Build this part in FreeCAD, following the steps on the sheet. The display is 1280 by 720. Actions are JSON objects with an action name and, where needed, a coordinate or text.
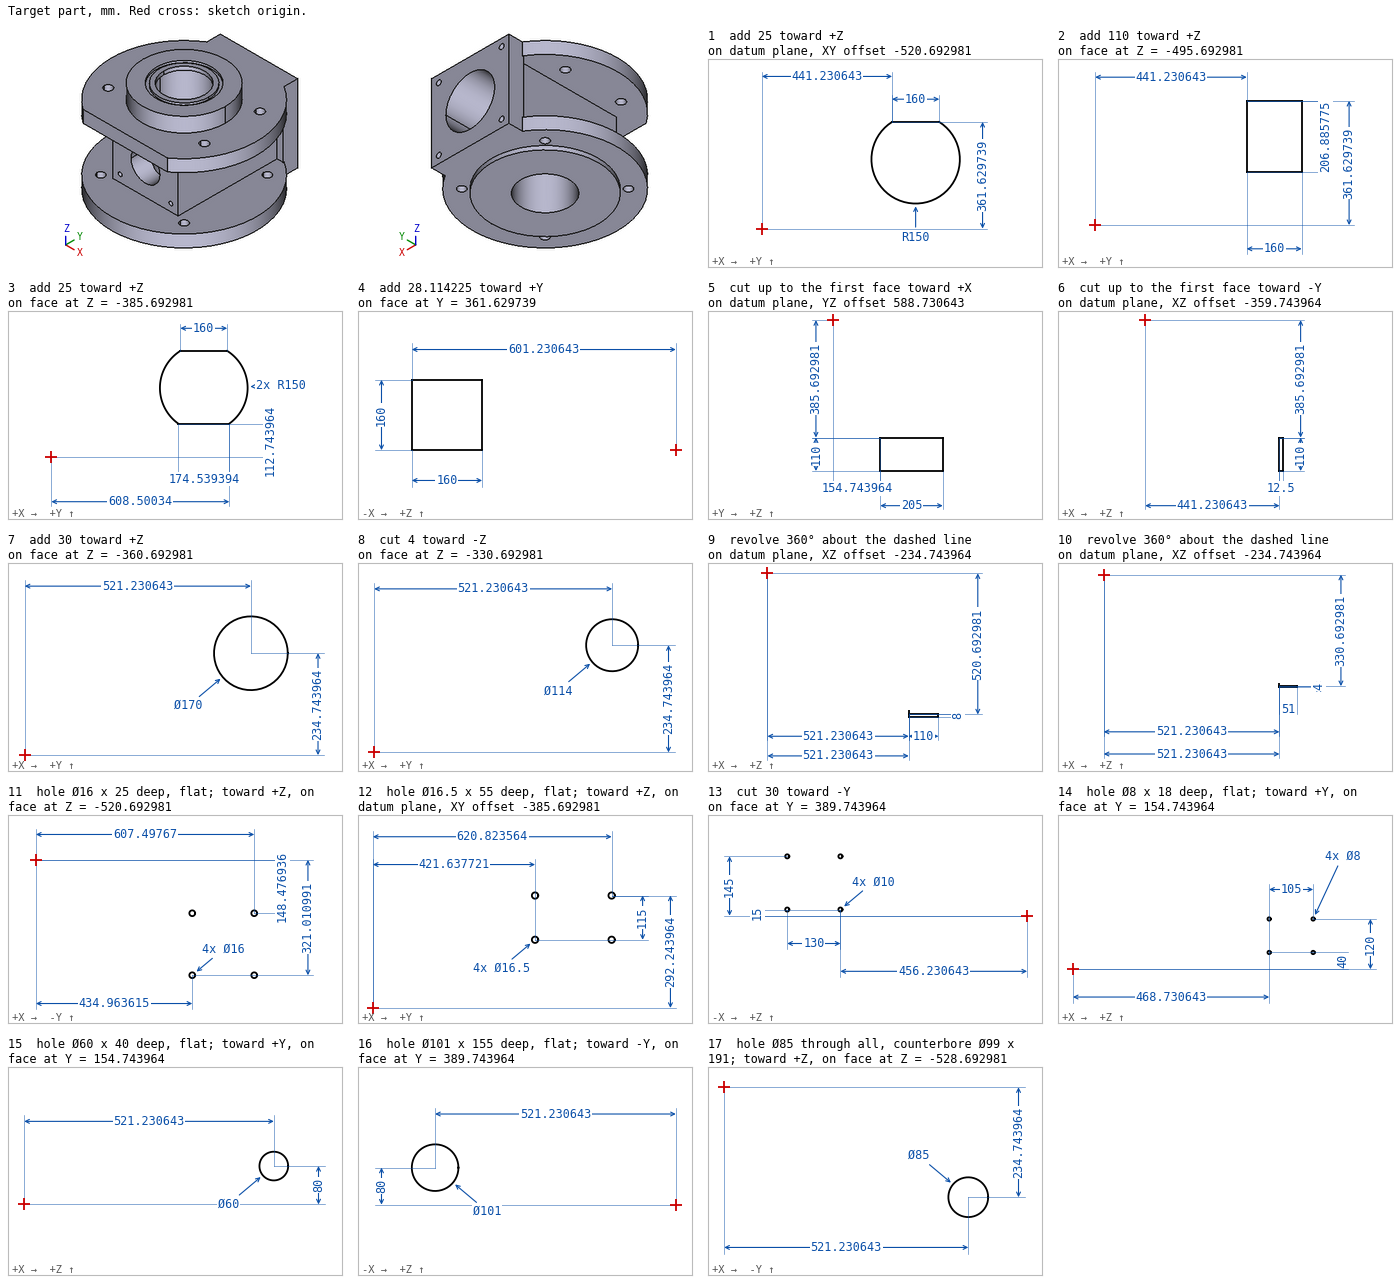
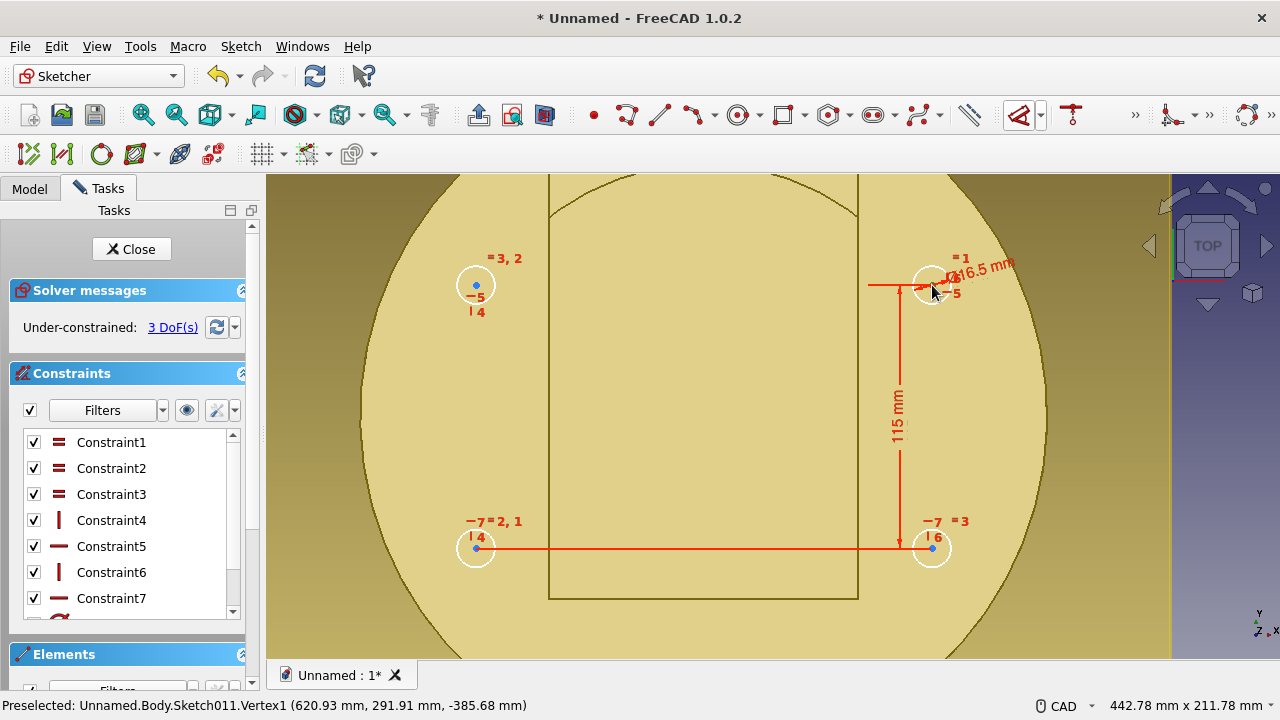
{"action": "key", "text": "l"}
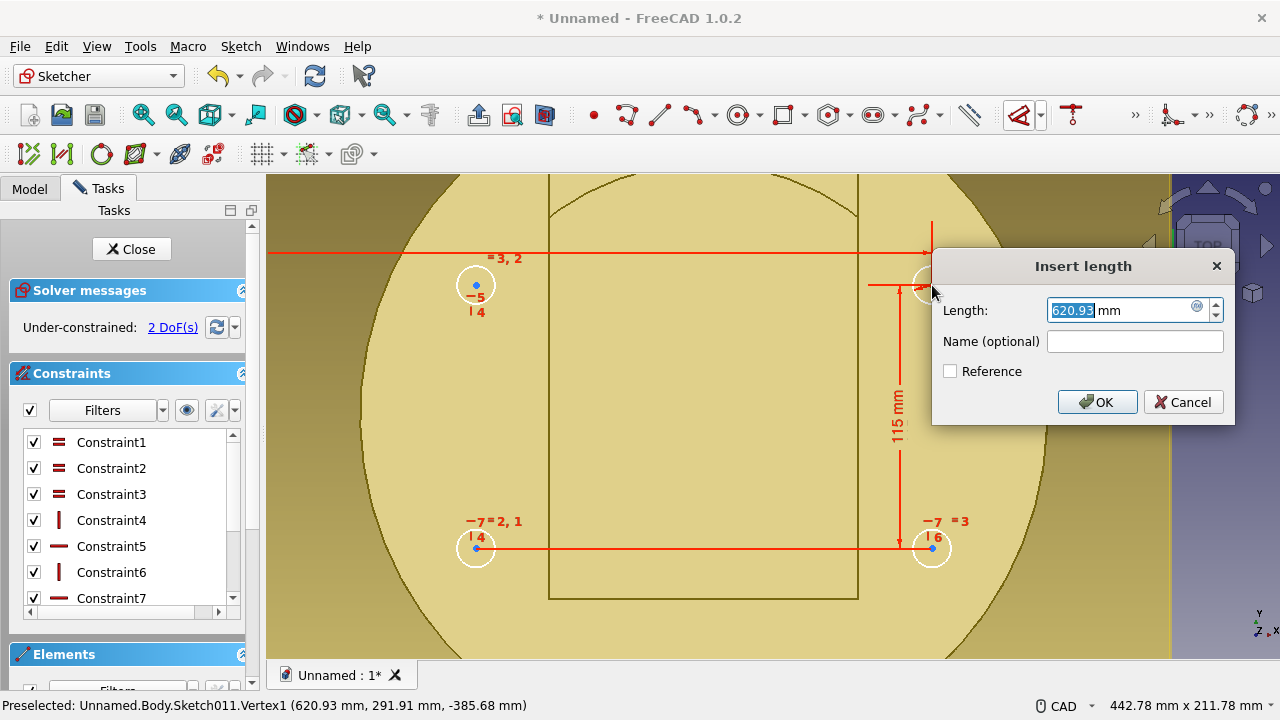
{"action": "type", "text": "620.823564"}
{"action": "key", "text": "Return"}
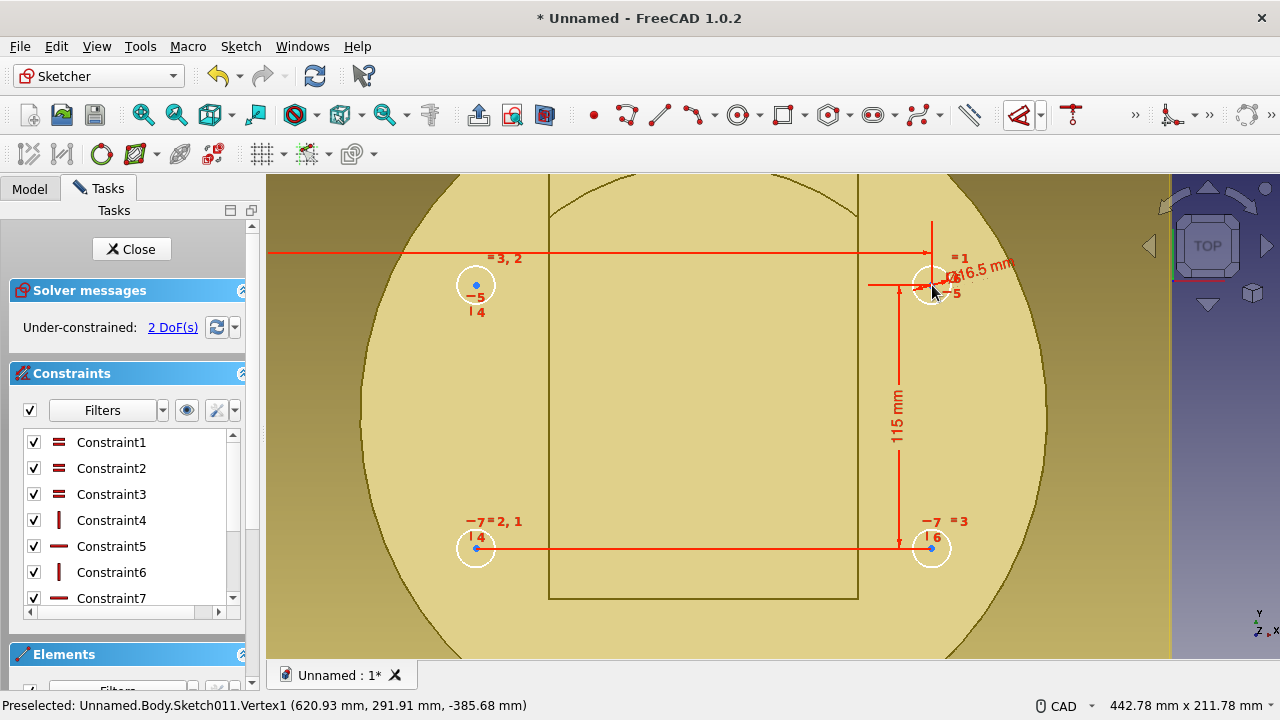
{"action": "left_click", "coordinate": [932, 285]}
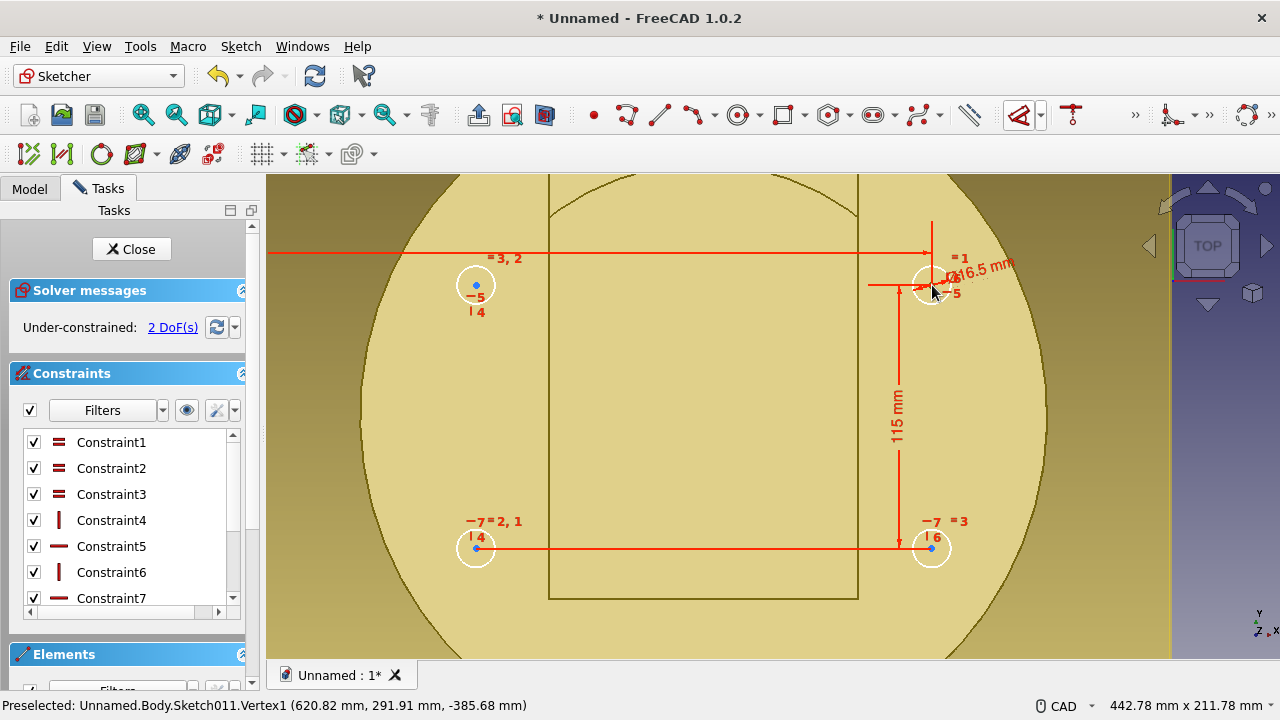
{"action": "key", "text": "i"}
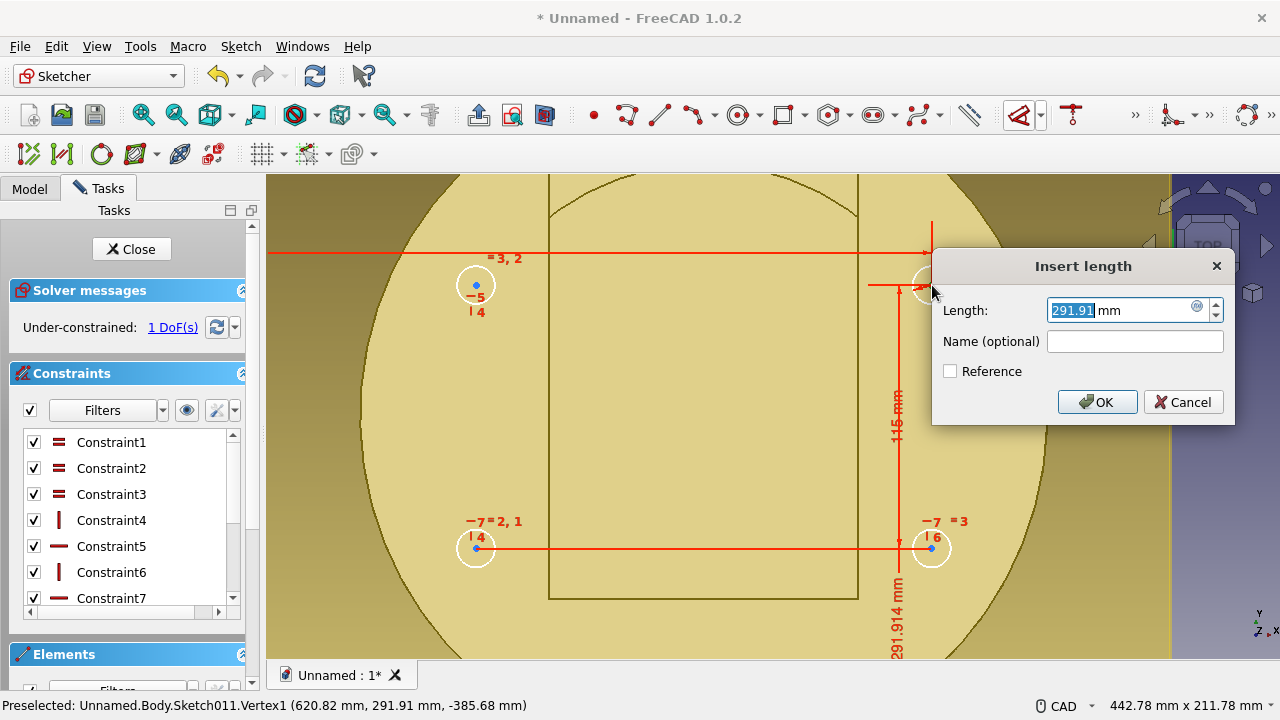
{"action": "type", "text": "292.243964"}
{"action": "key", "text": "Return"}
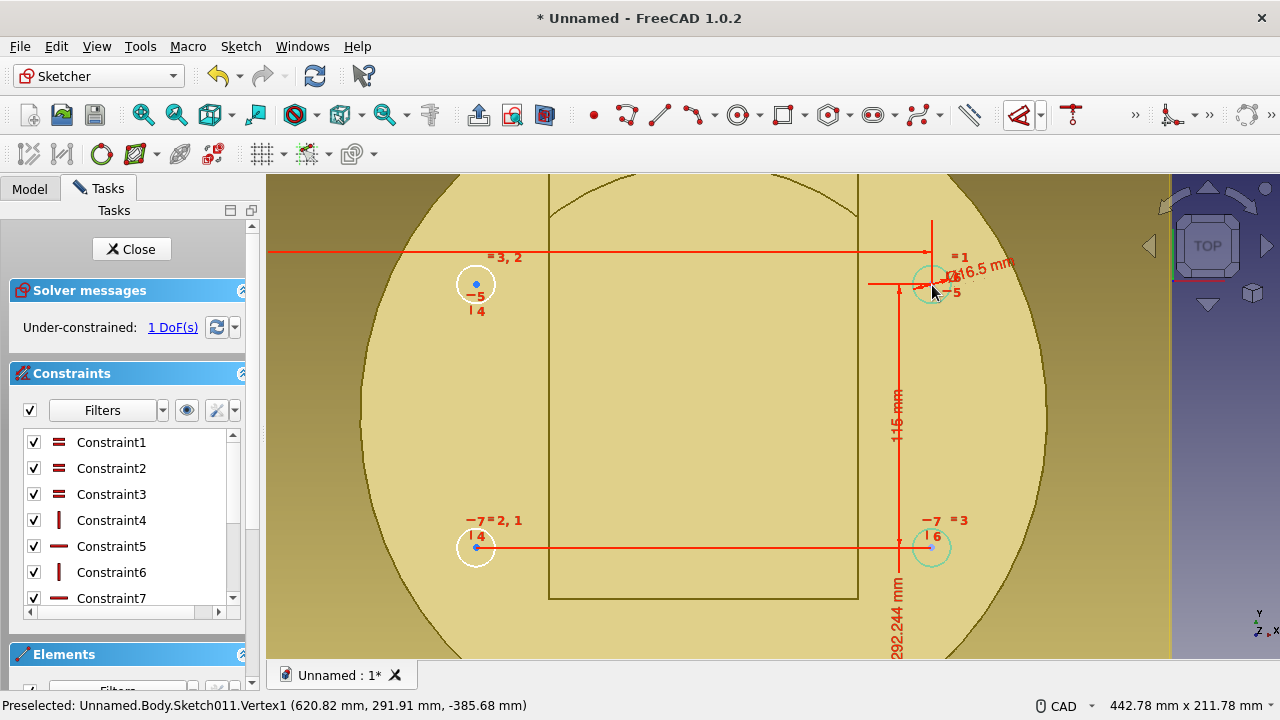
{"action": "left_click", "coordinate": [476, 548]}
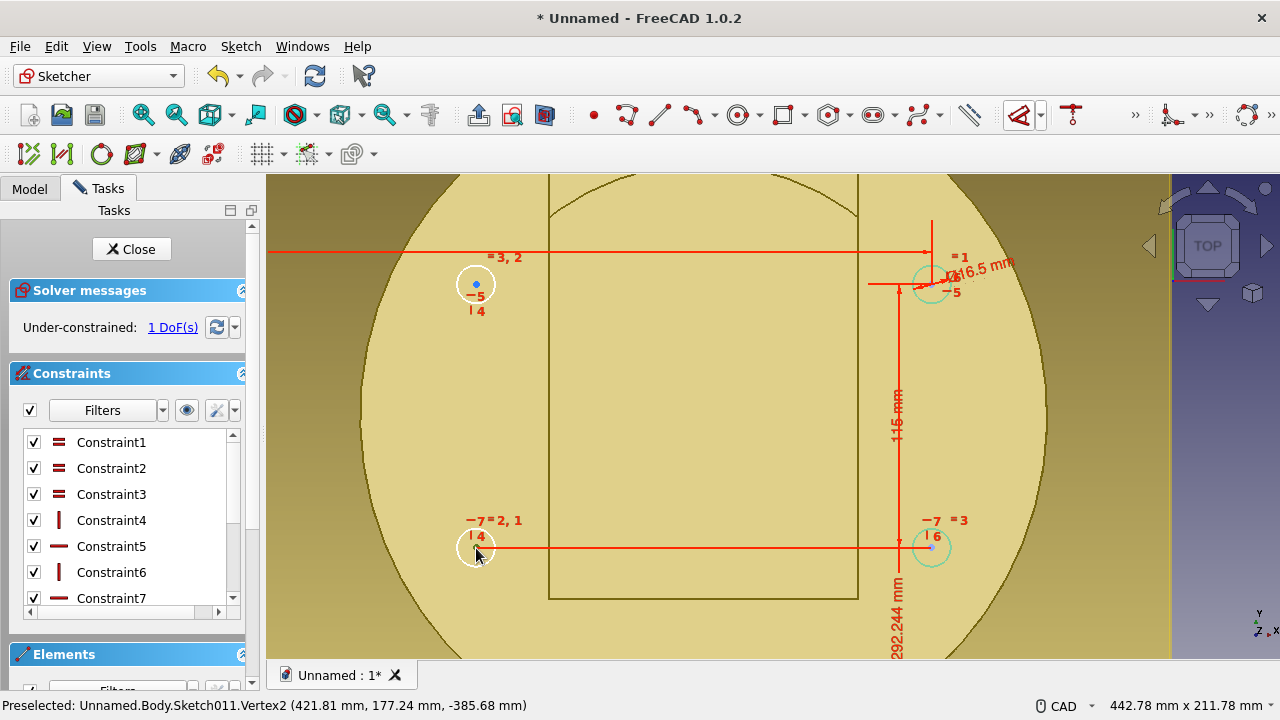
{"action": "left_click", "coordinate": [1040, 116]}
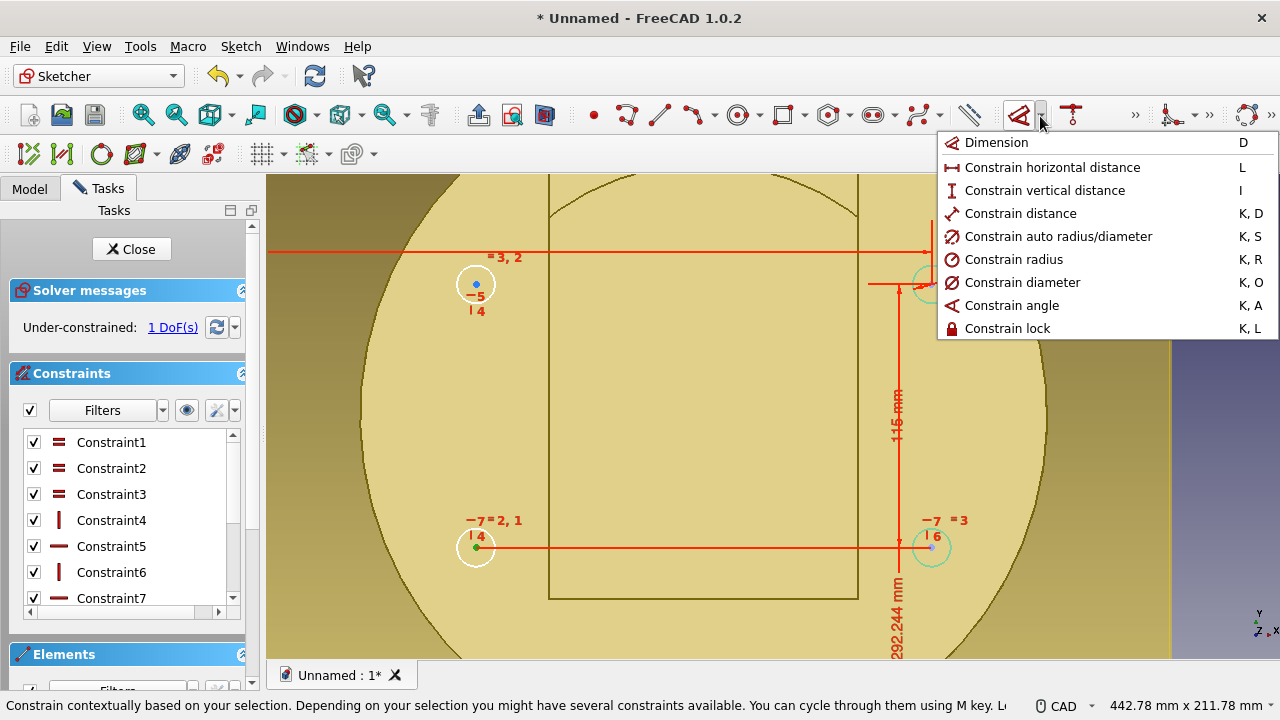
{"action": "left_click", "coordinate": [1108, 168]}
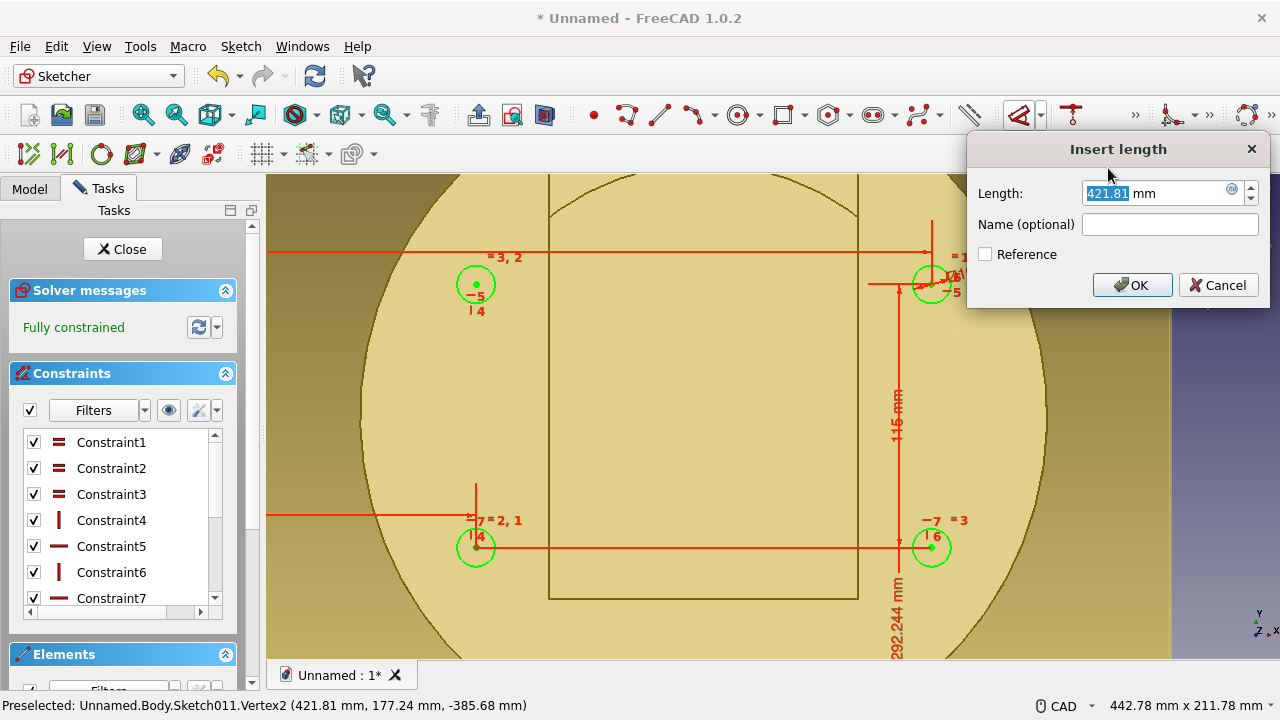
{"action": "type", "text": "421.637721"}
{"action": "key", "text": "Return"}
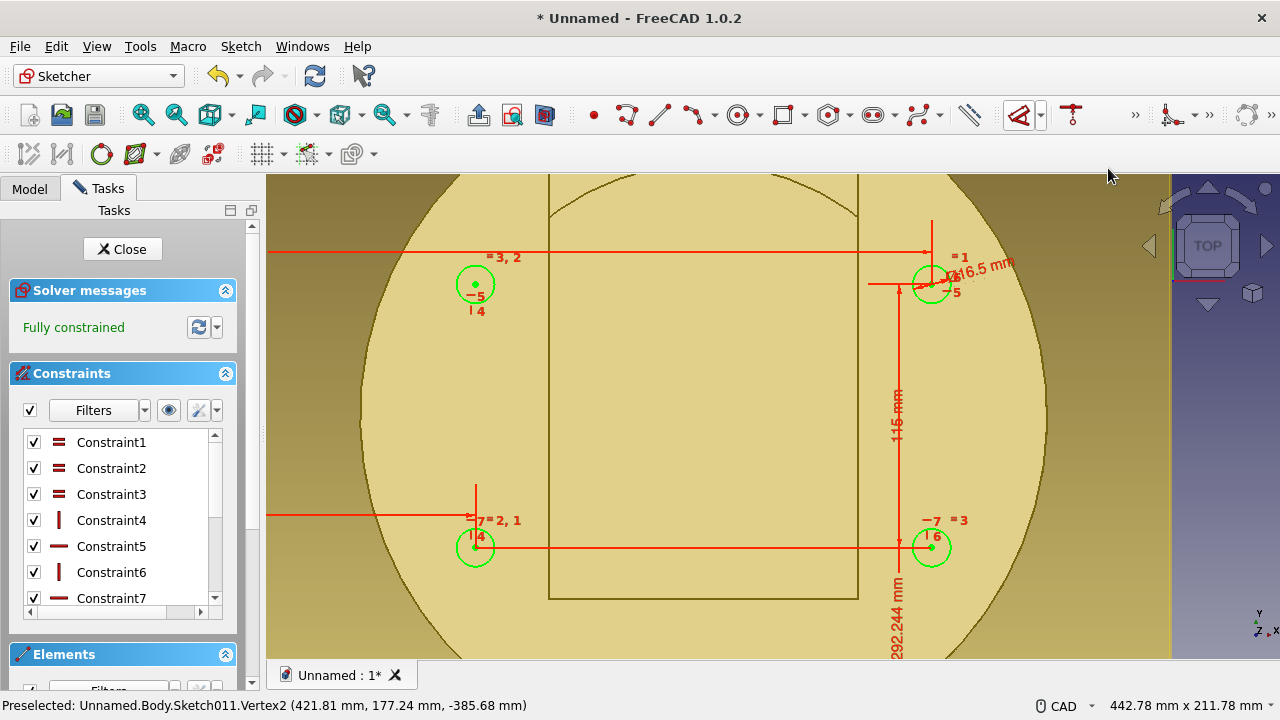
{"action": "left_click", "coordinate": [123, 249]}